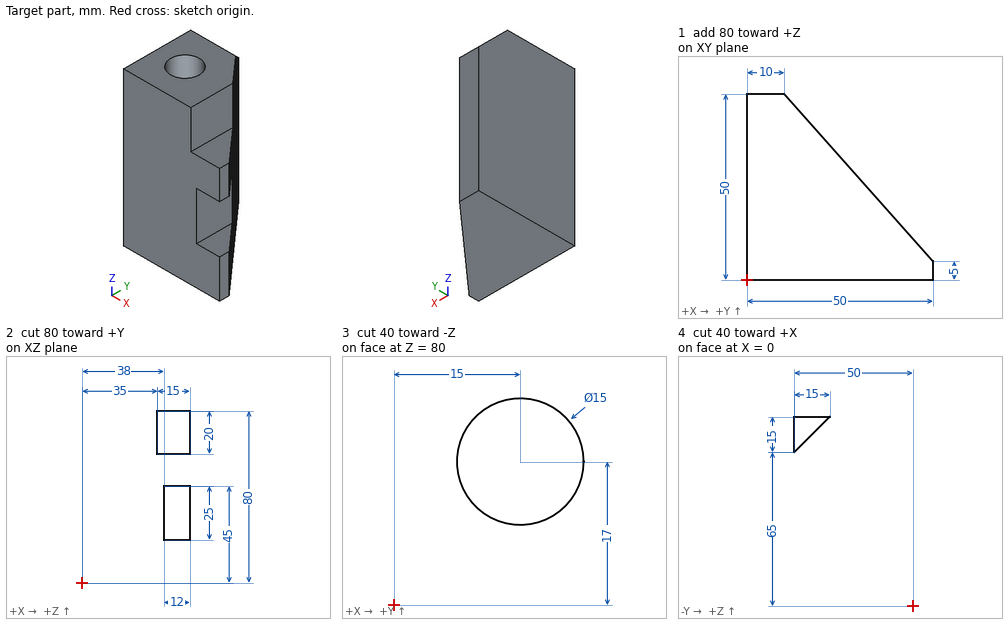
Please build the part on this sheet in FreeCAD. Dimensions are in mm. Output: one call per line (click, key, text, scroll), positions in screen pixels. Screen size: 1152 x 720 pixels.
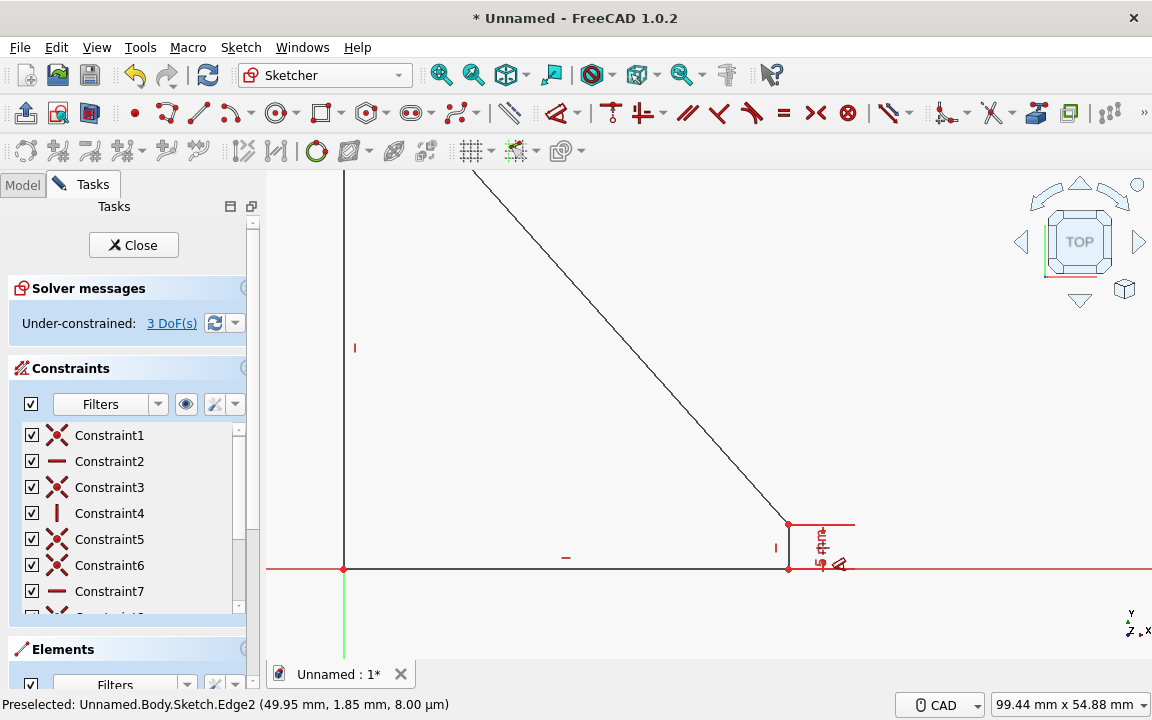
click(477, 569)
click(566, 603)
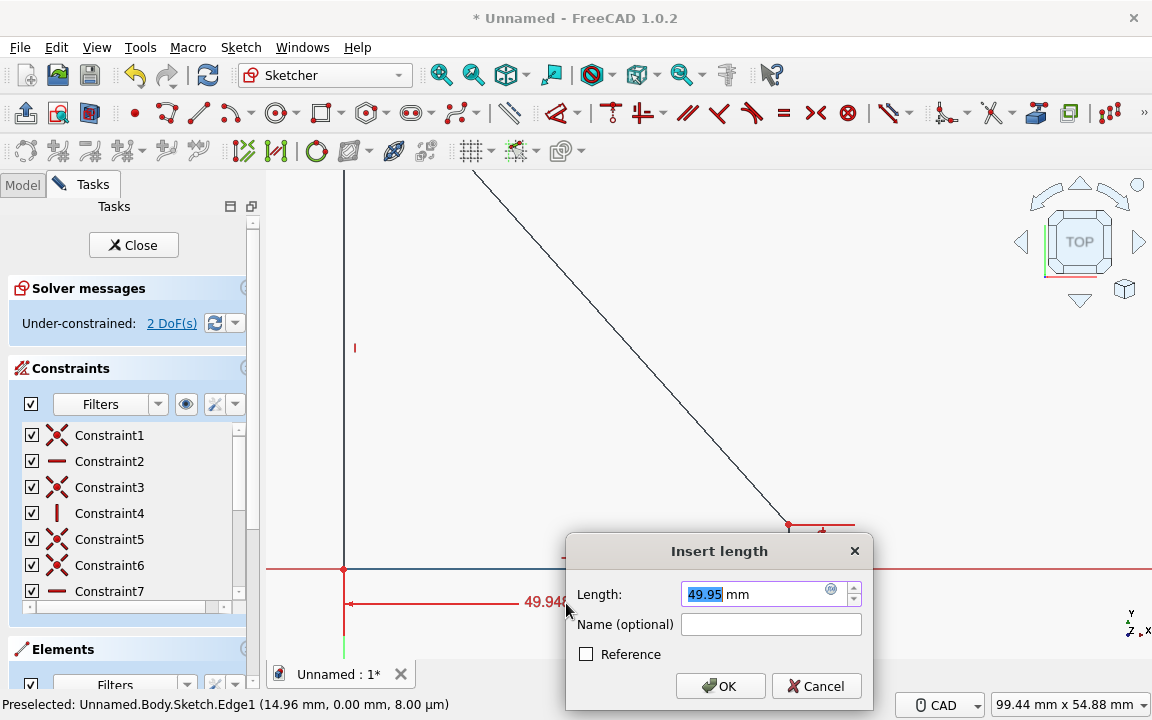
text(50)
key(Return)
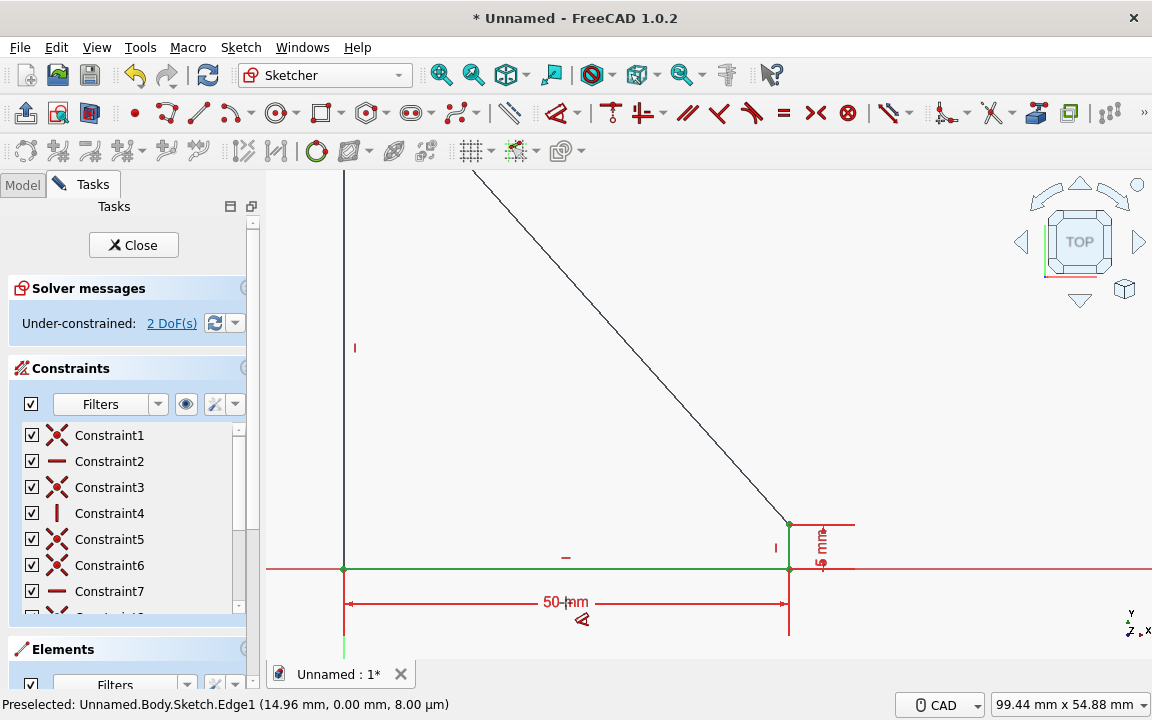
scroll(791, 552, down, 2)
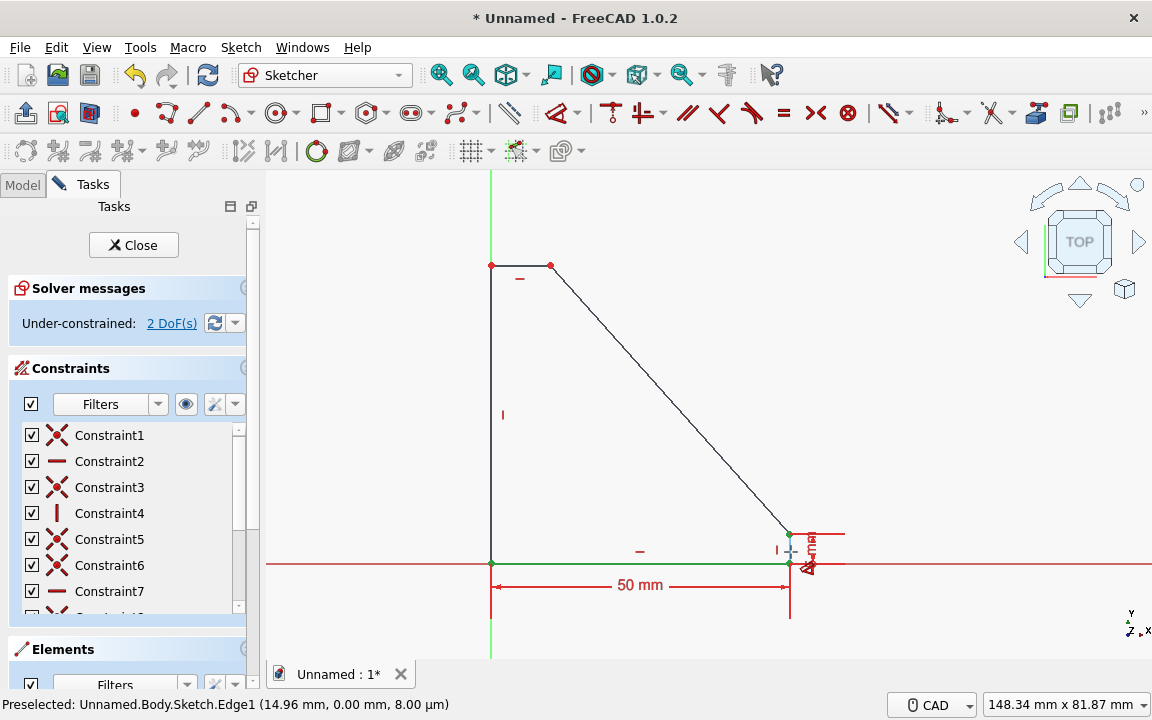
click(533, 266)
click(521, 232)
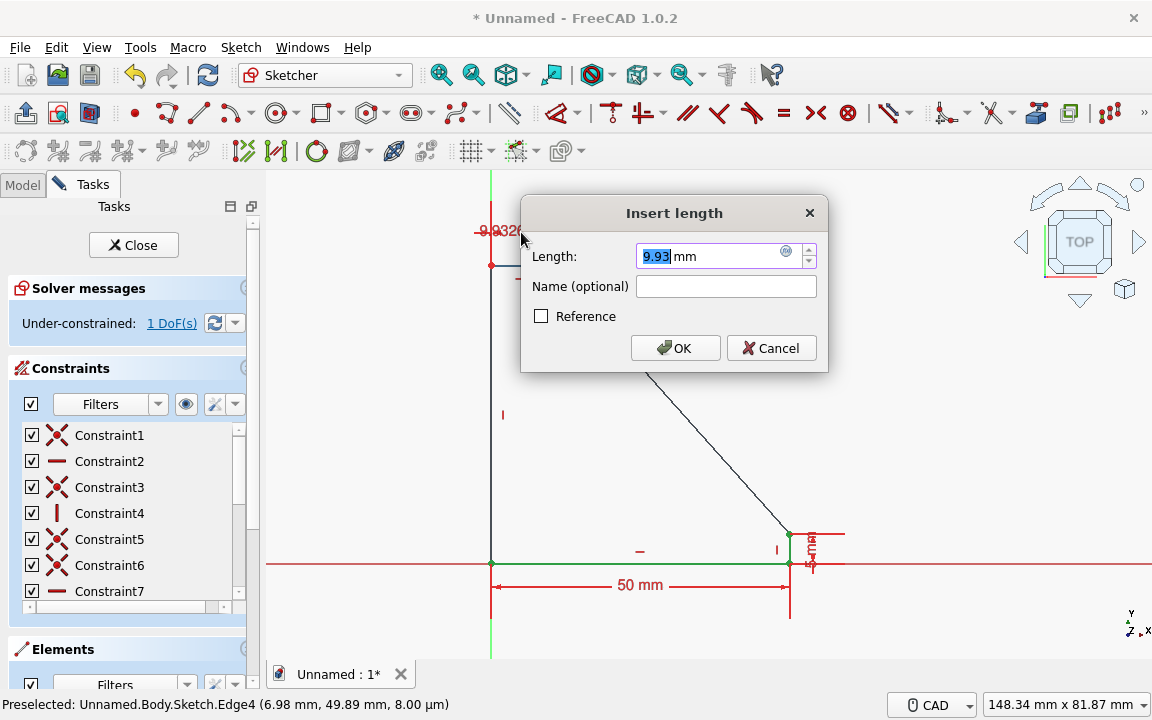
text(10)
key(Return)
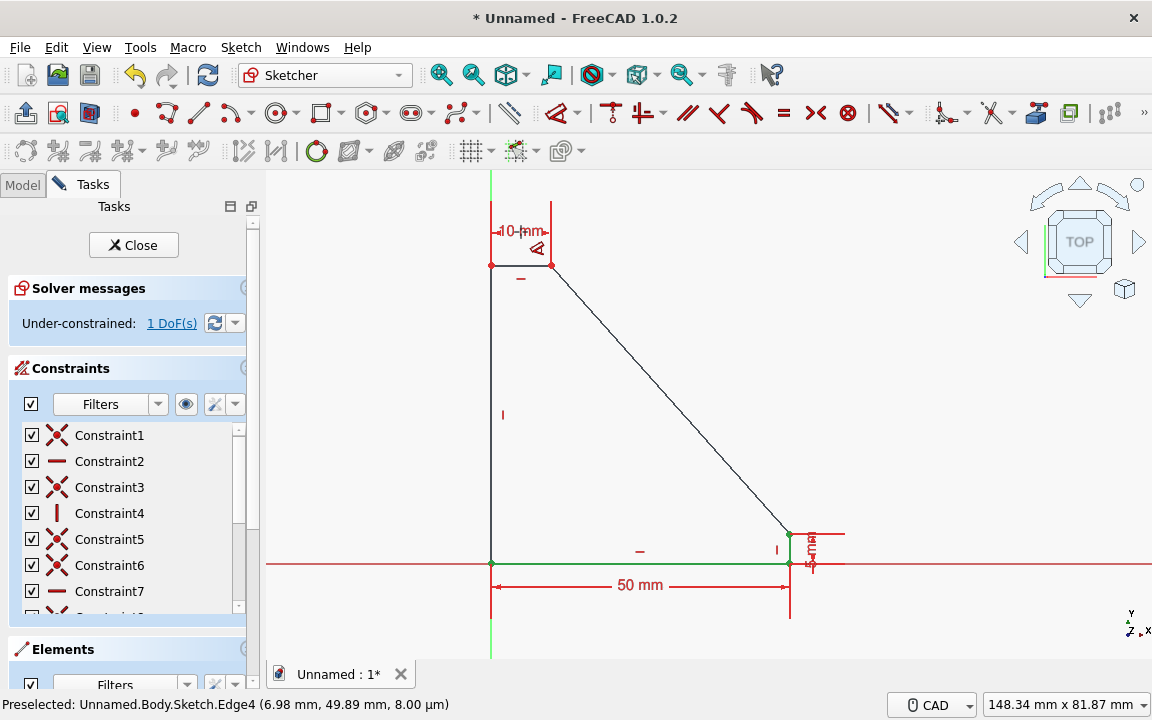
click(491, 355)
click(457, 415)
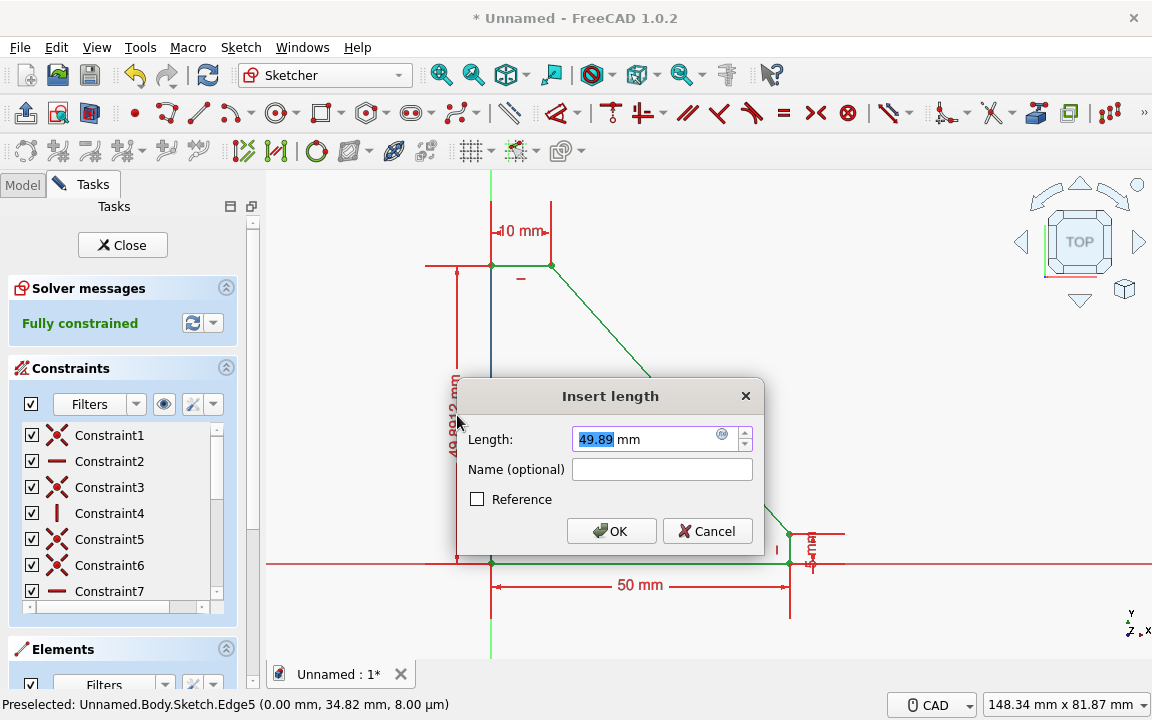
text(50)
key(Return)
key(Escape)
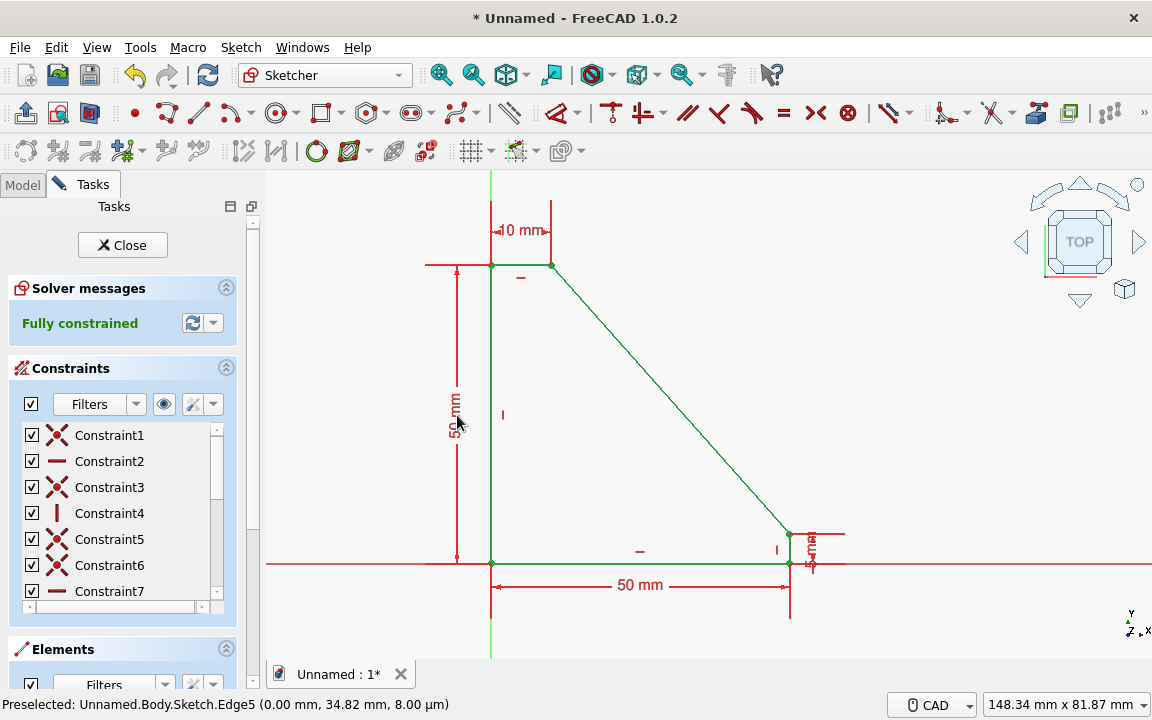
click(123, 245)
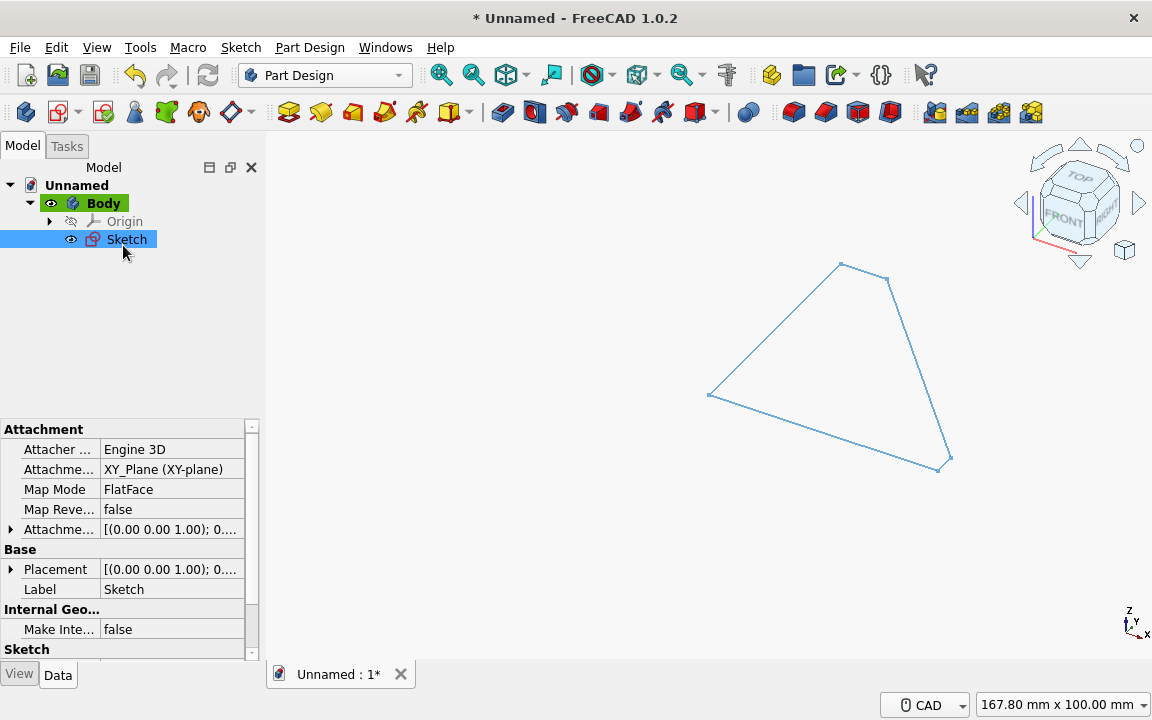
click(290, 112)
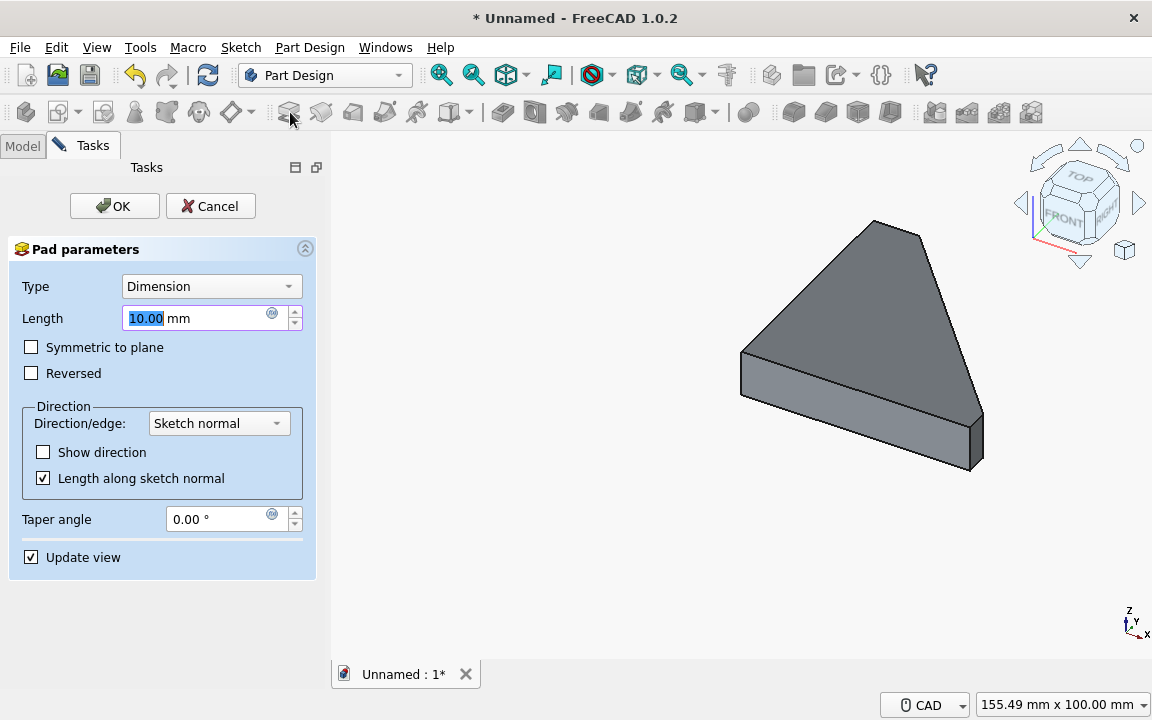
text(80)
key(Tab)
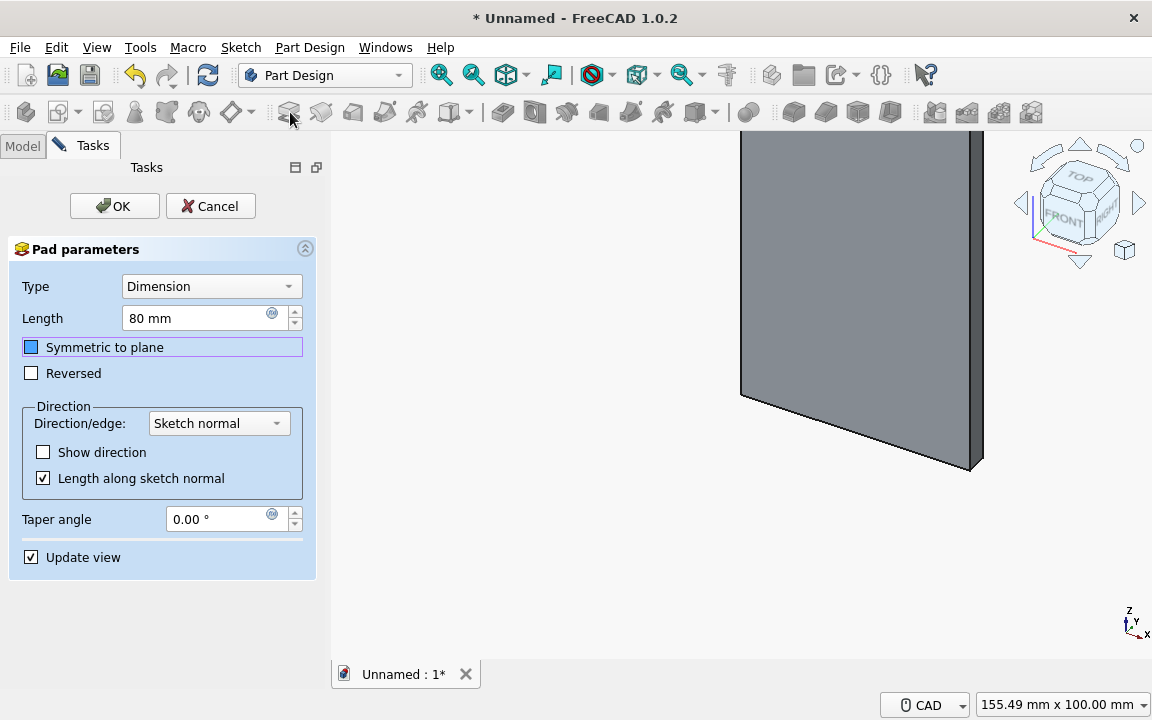
click(115, 206)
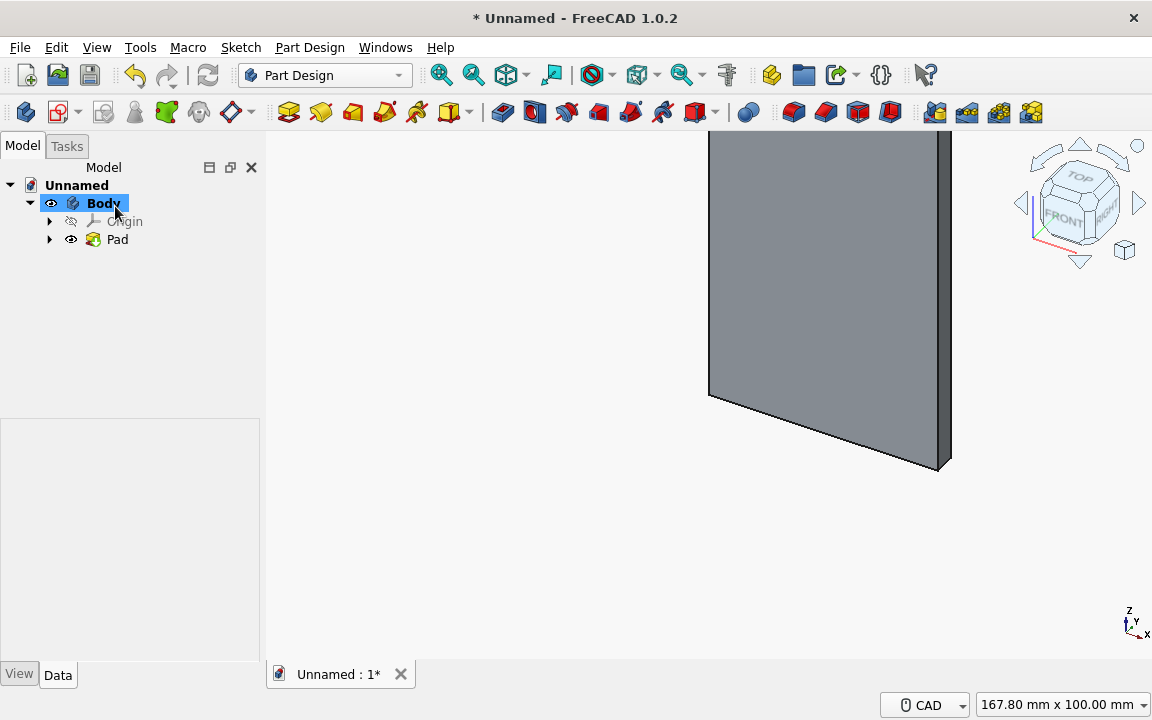
click(442, 76)